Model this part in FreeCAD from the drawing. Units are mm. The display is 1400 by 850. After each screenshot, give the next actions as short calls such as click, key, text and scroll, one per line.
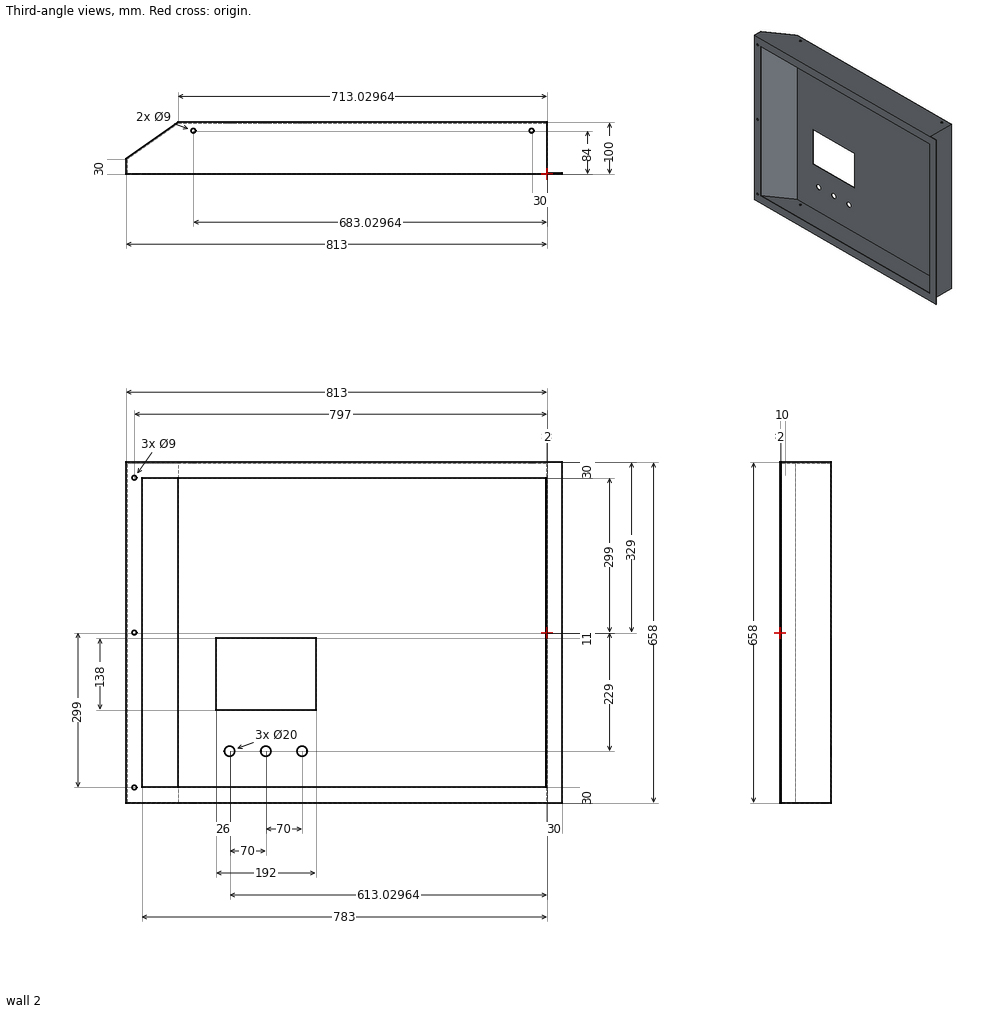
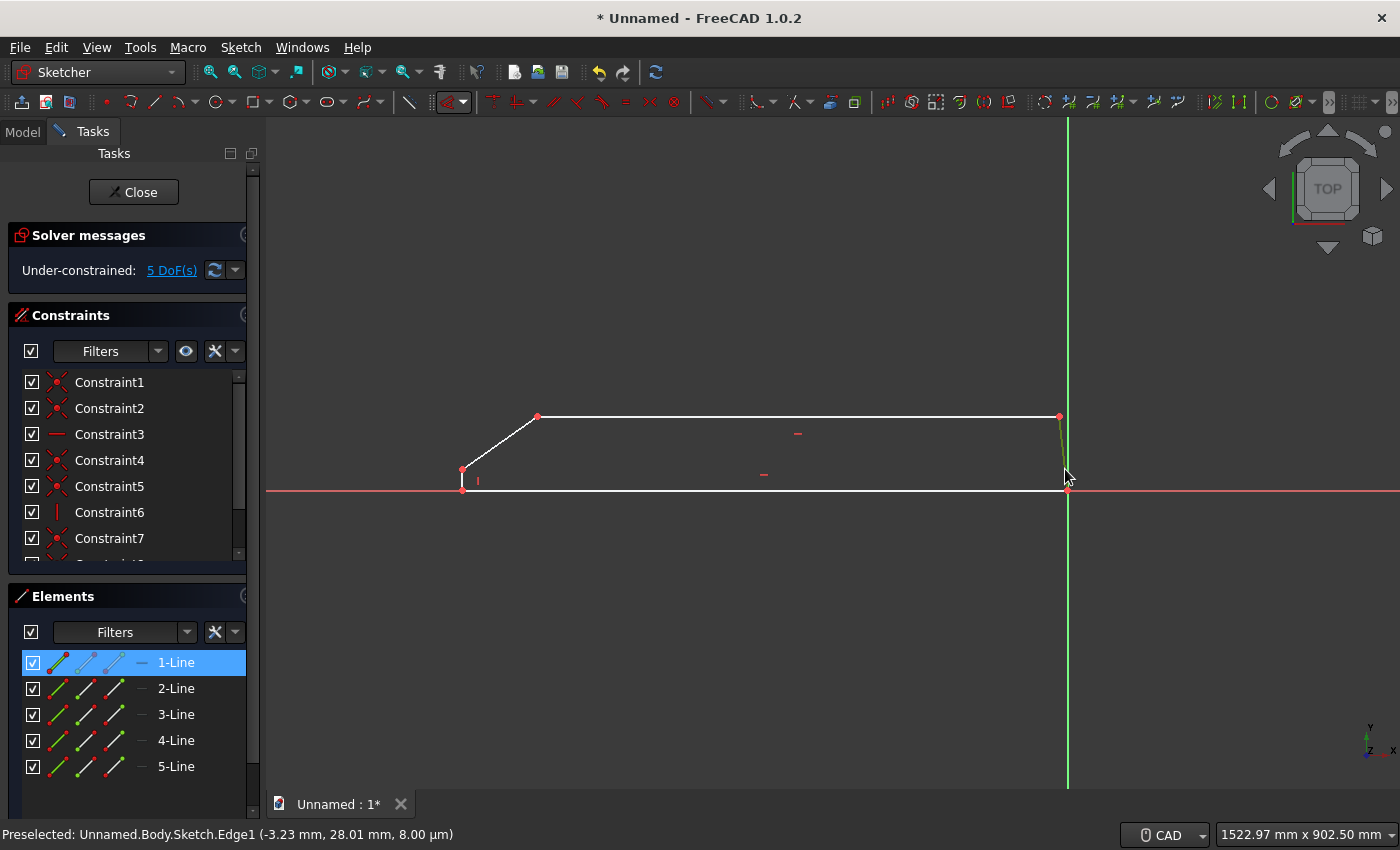
click(536, 102)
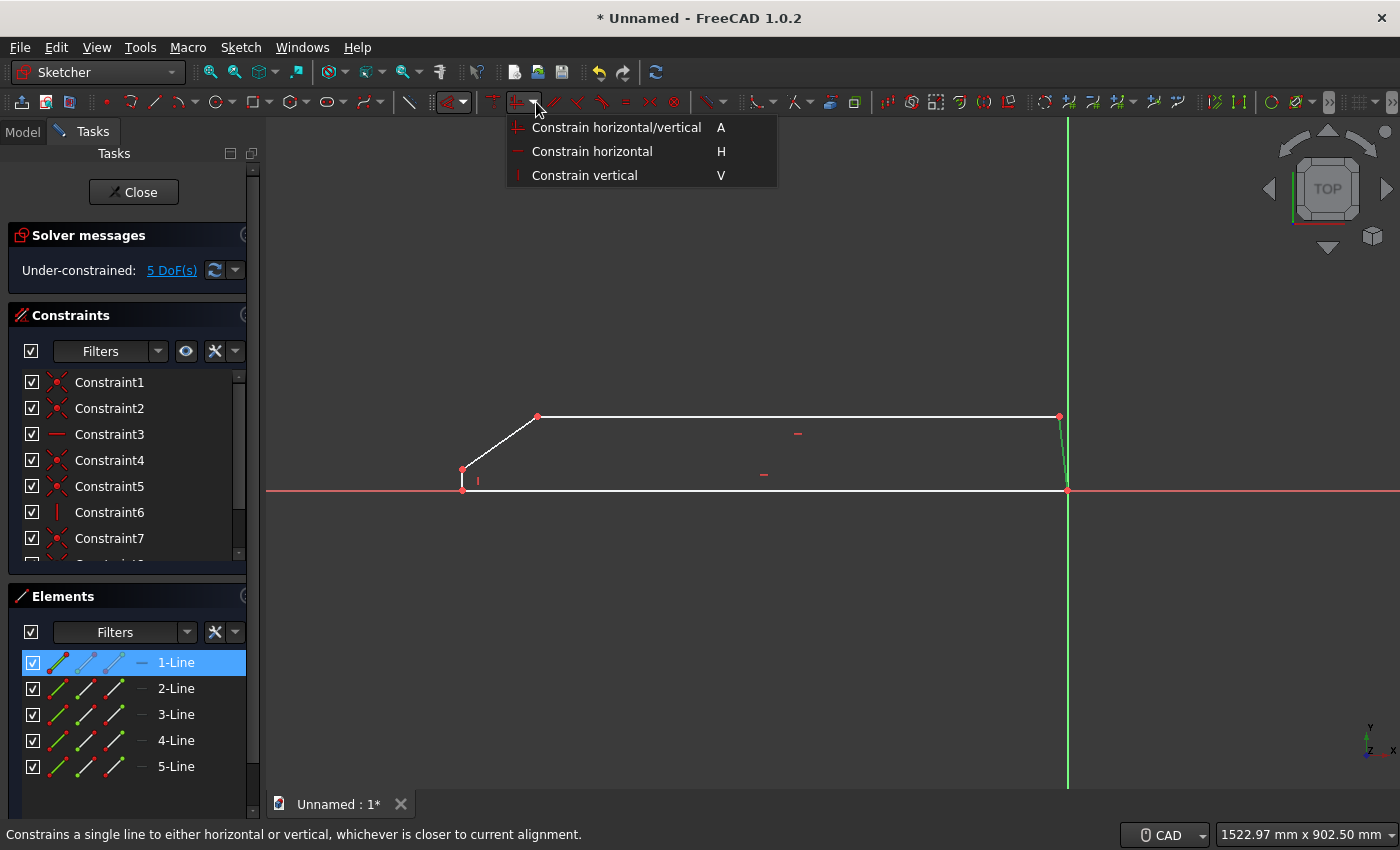
click(642, 175)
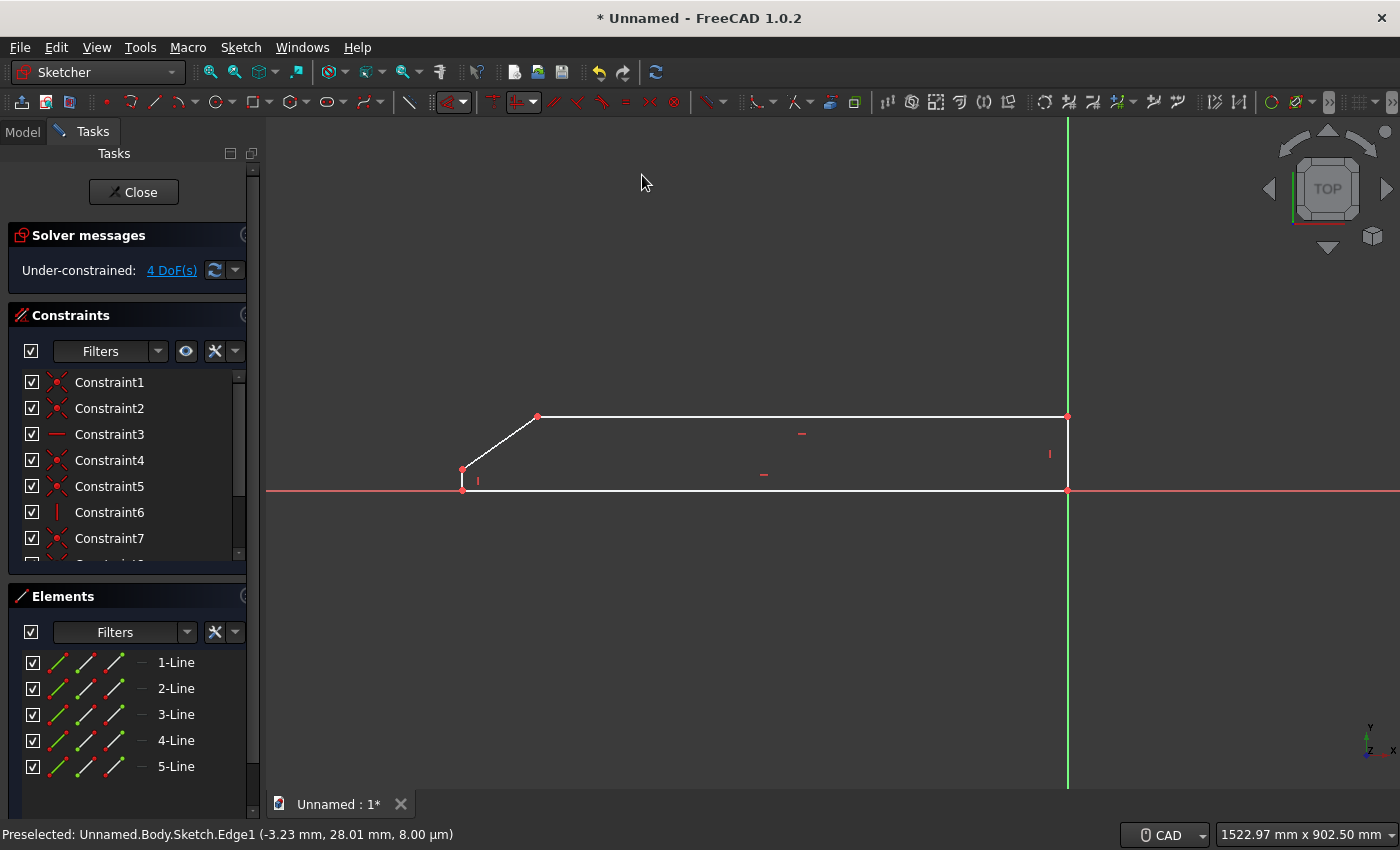
click(448, 102)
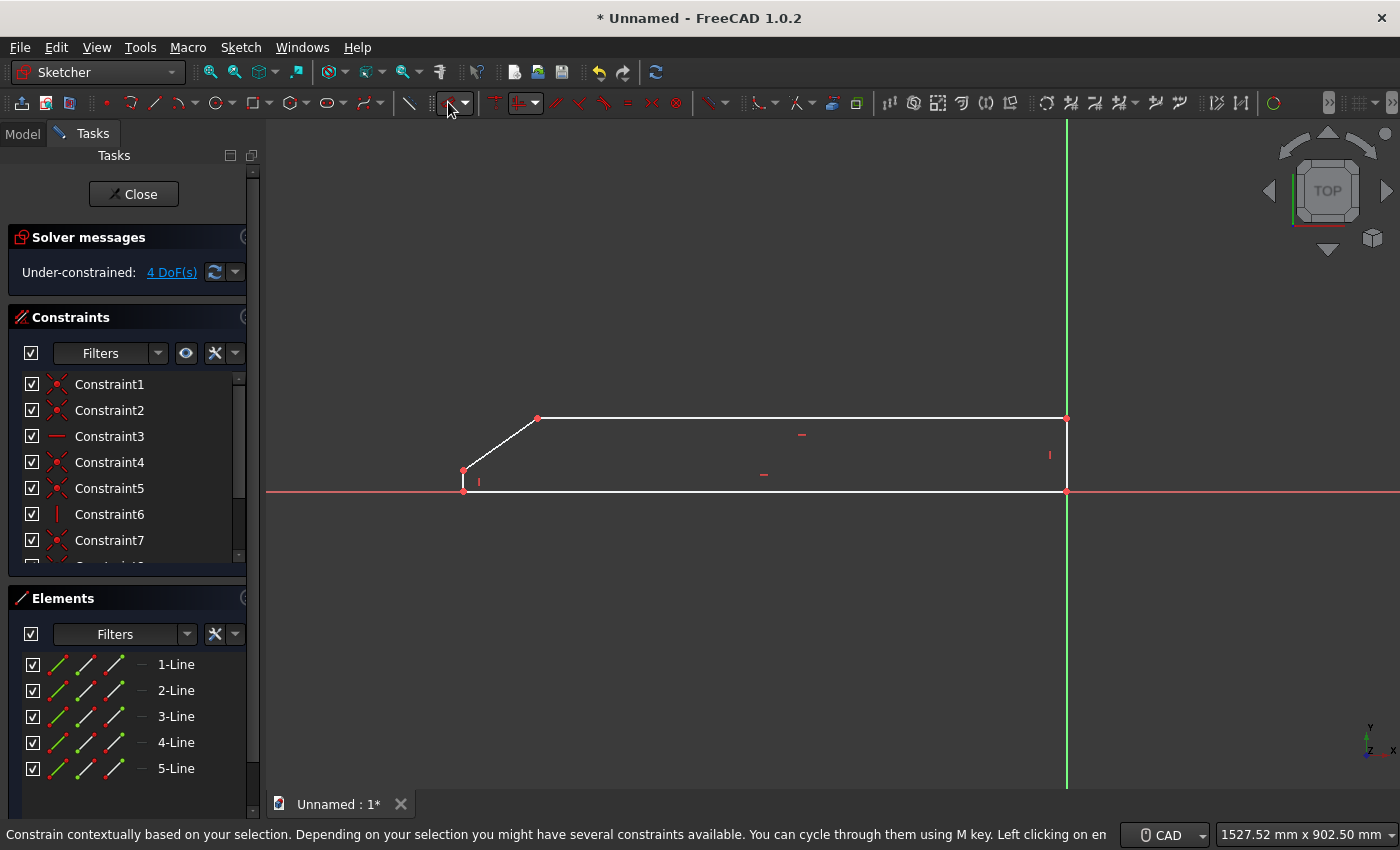
scroll(463, 481, up, 3)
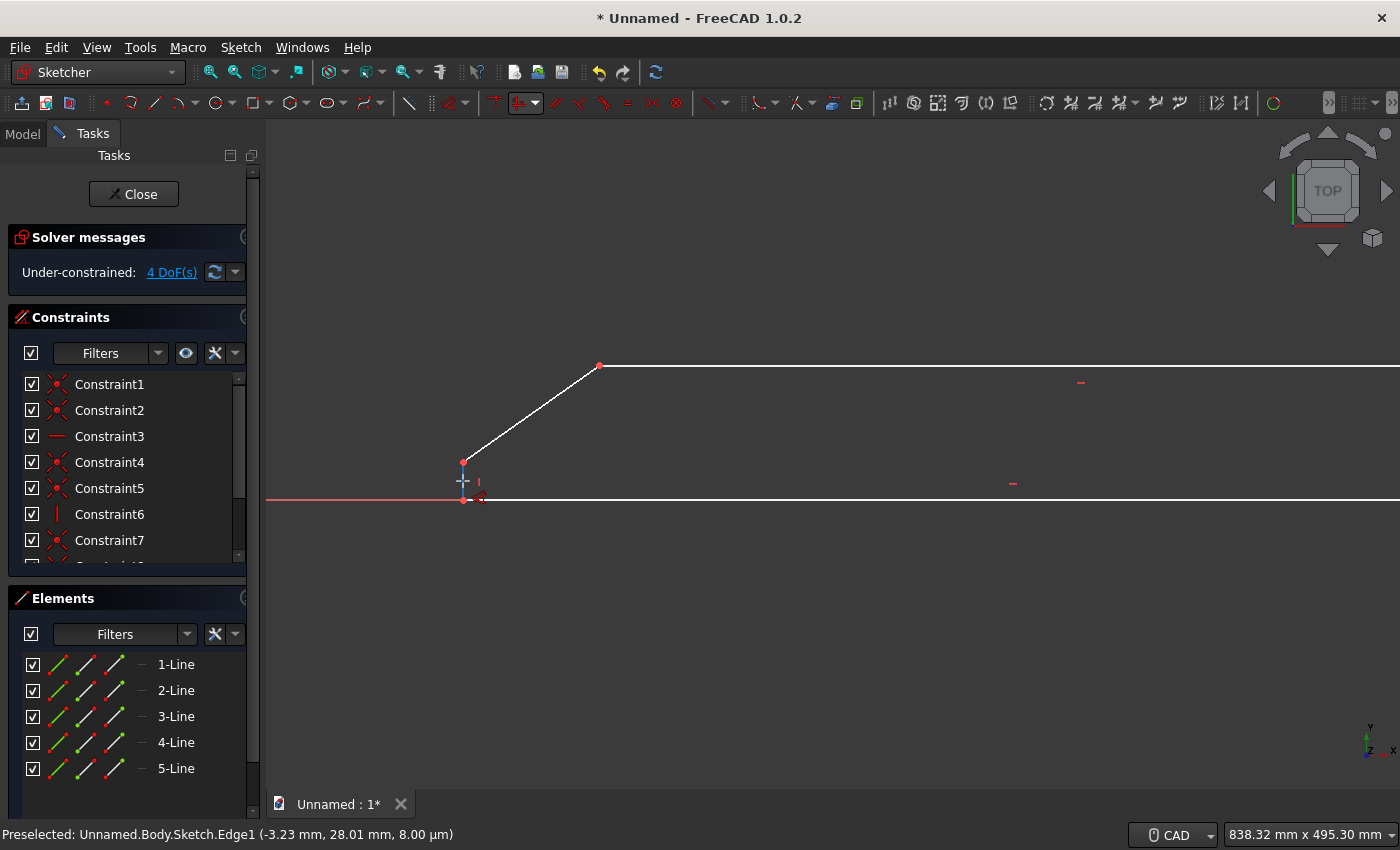
click(463, 481)
click(429, 481)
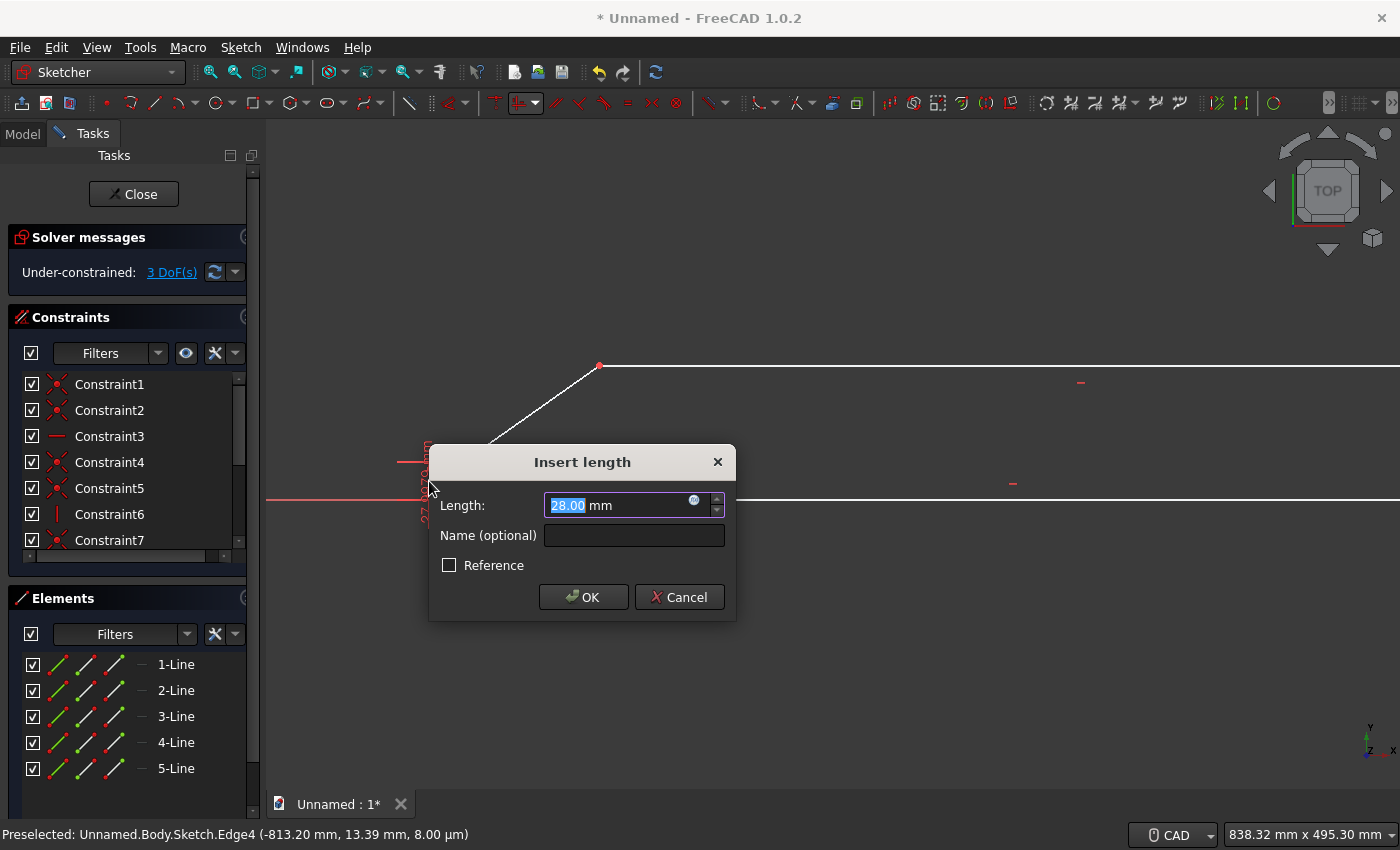
text(30)
key(Return)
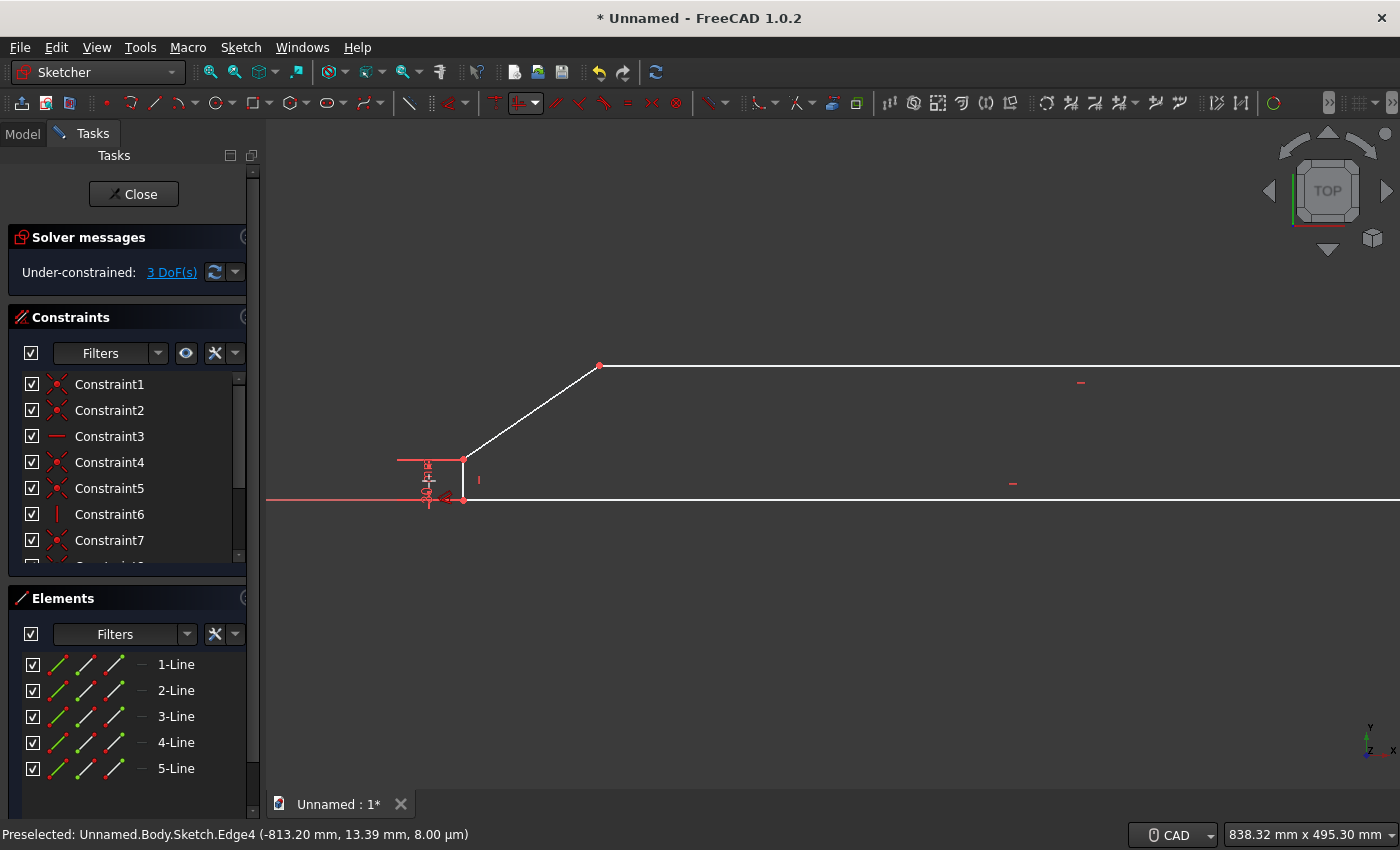
scroll(462, 480, down, 3)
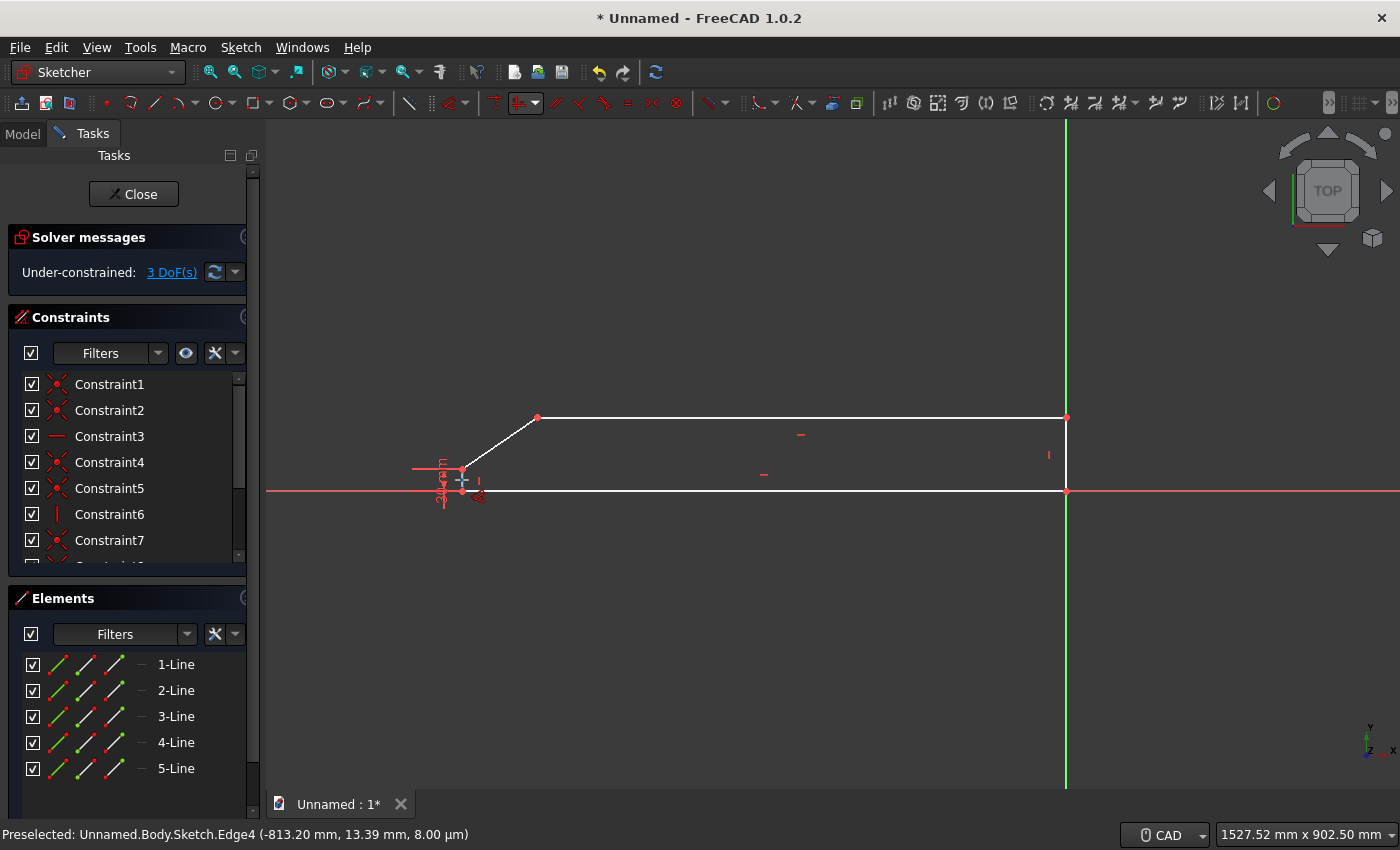
click(1066, 469)
click(1100, 454)